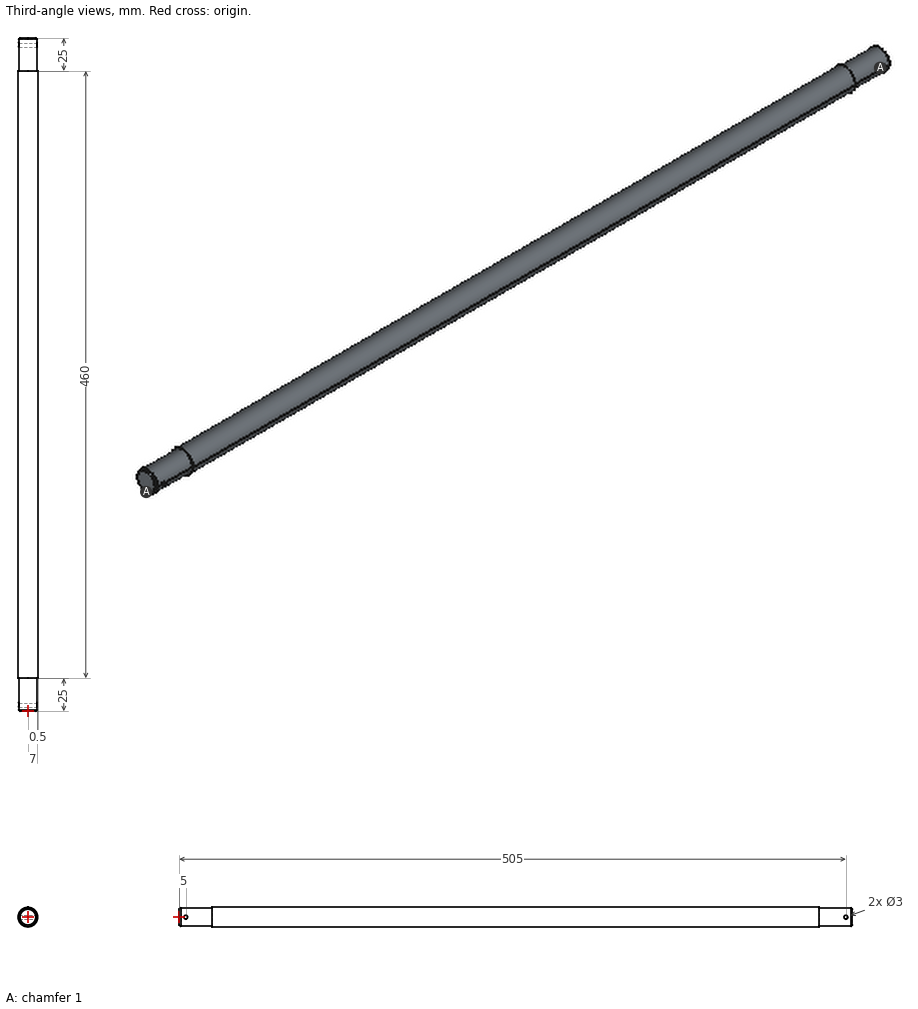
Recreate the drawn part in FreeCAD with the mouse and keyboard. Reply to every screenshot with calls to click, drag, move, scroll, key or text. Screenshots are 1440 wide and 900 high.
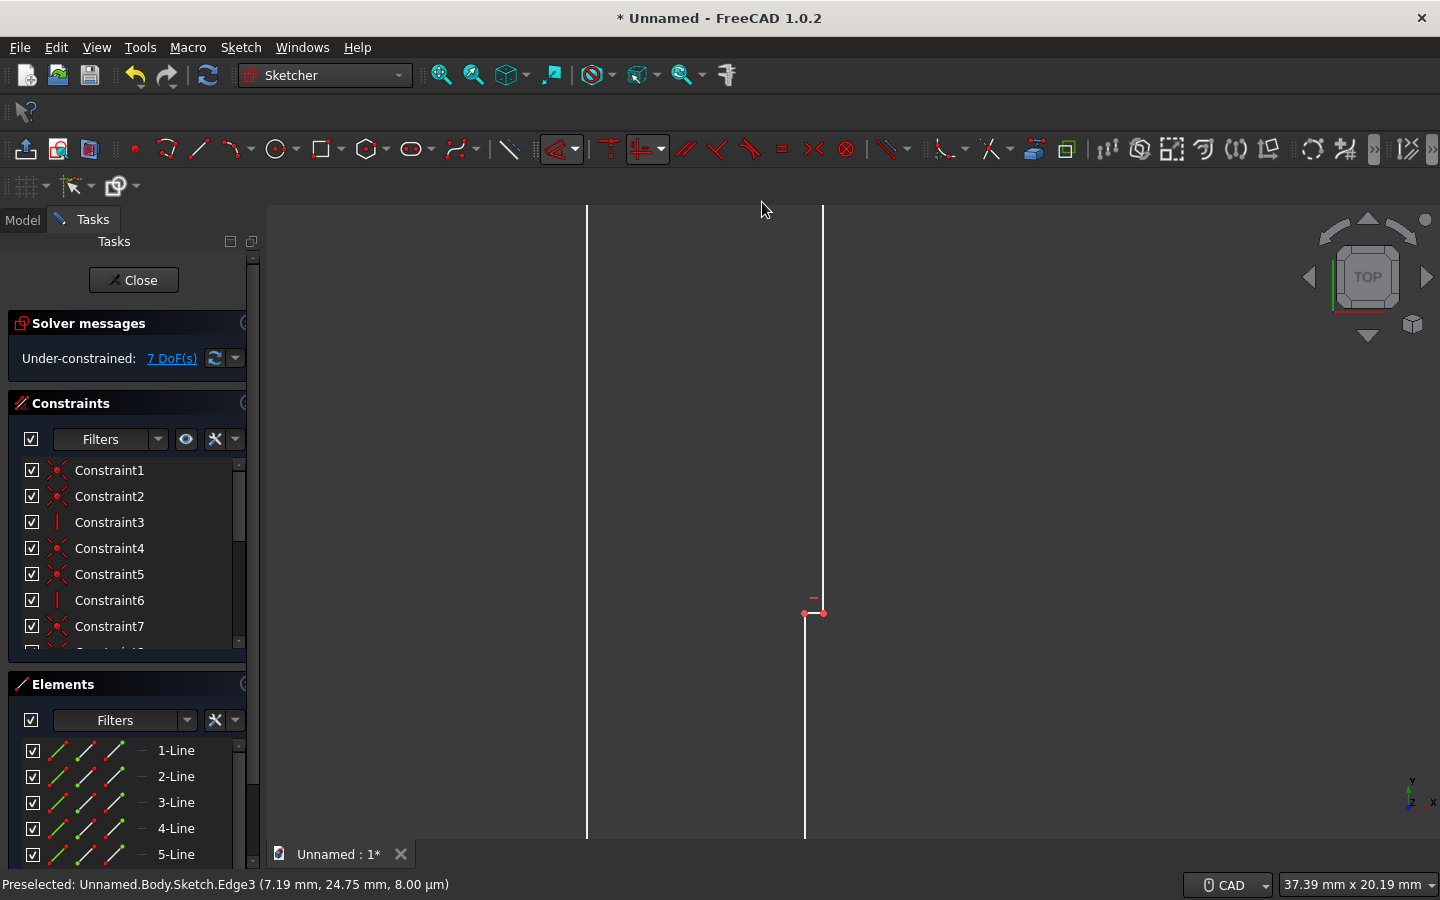
scroll(787, 723, down, 18)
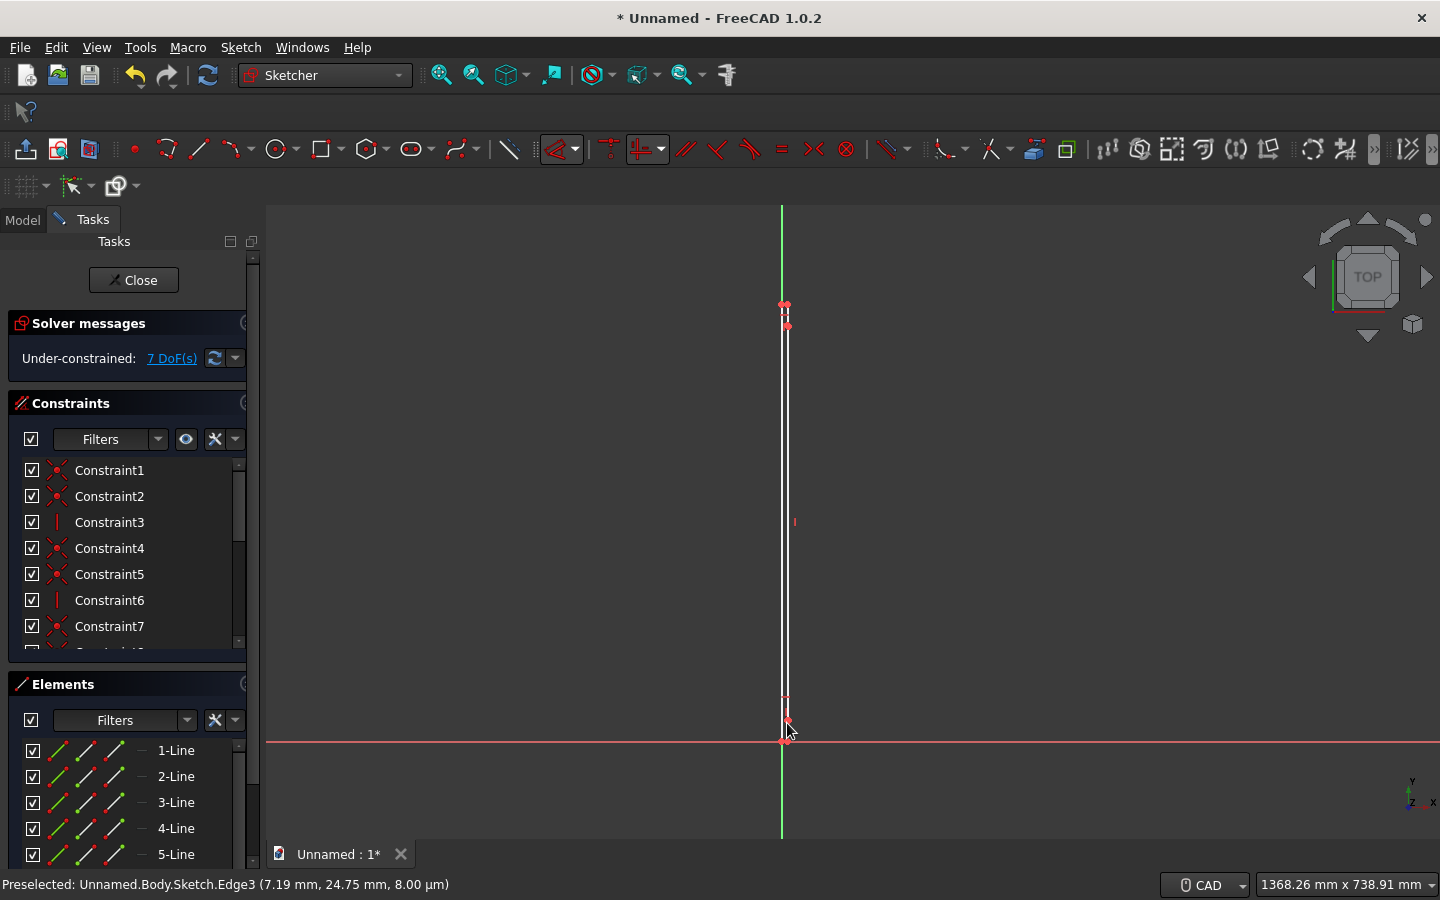
scroll(788, 326, up, 14)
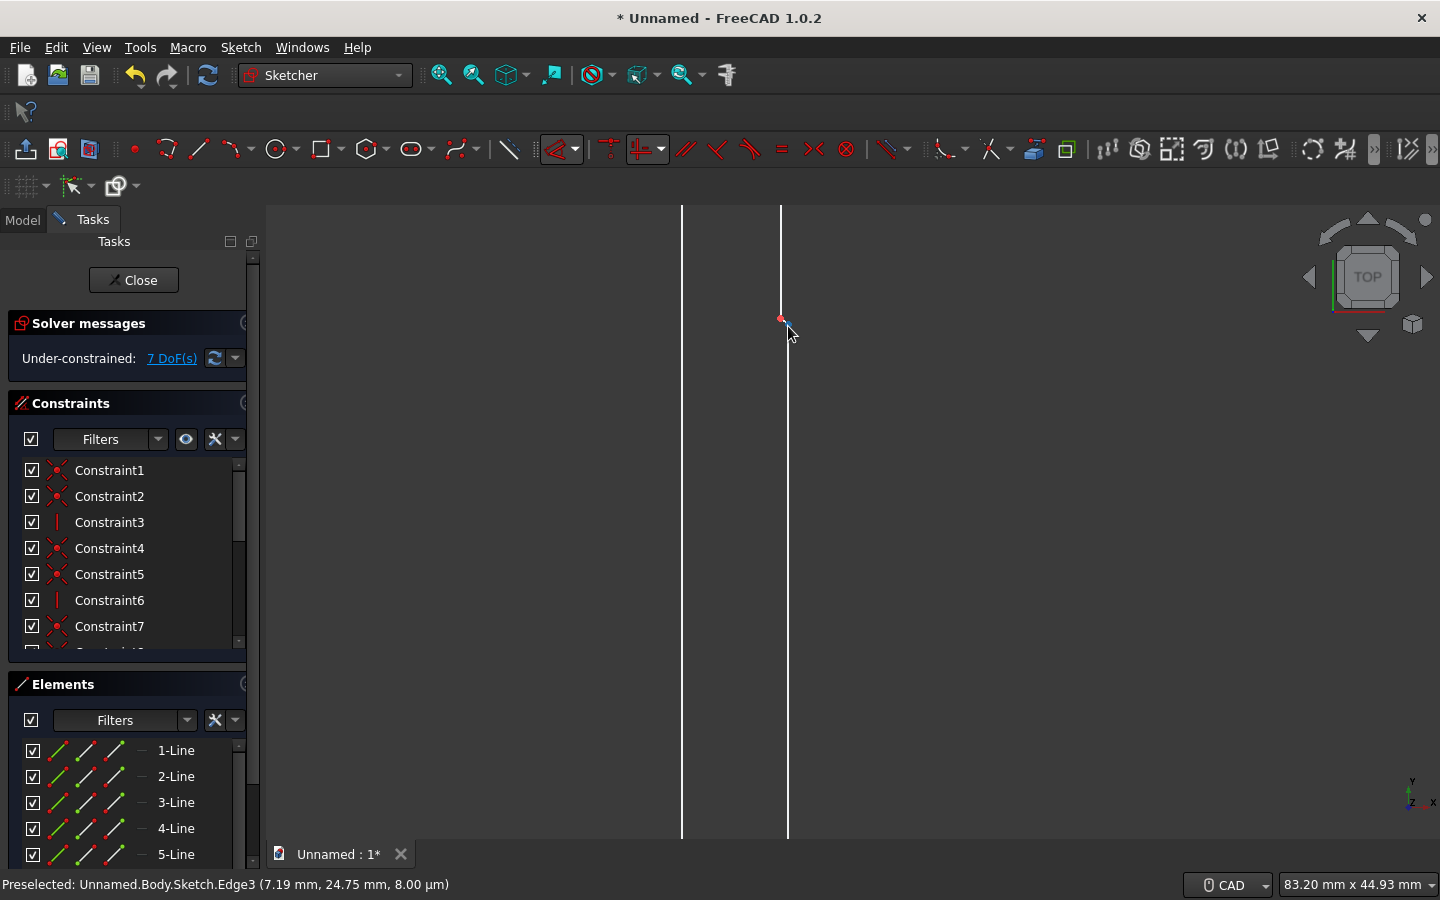
scroll(784, 321, up, 4)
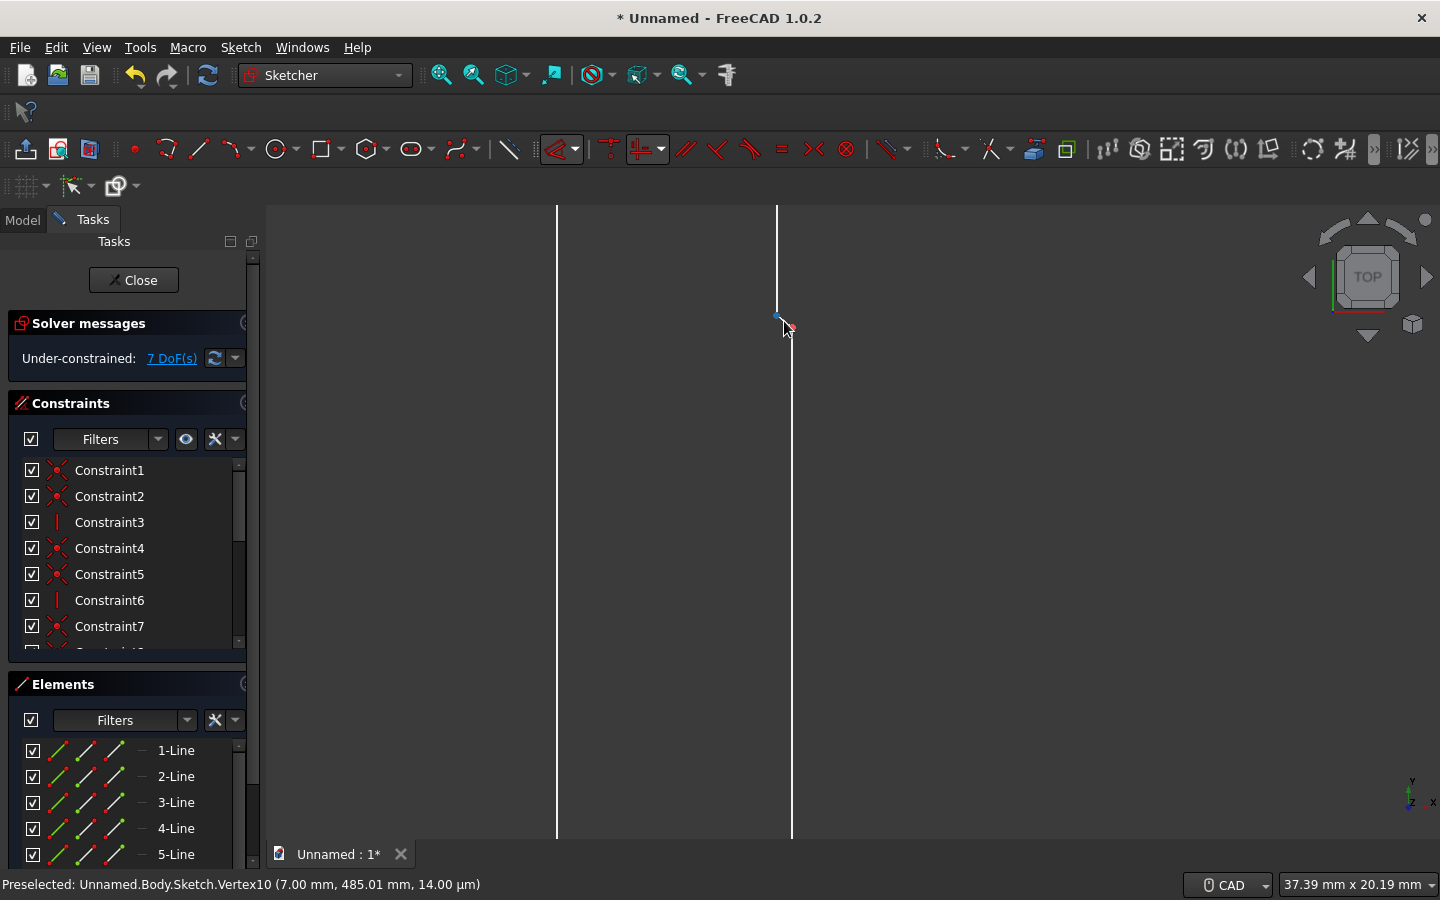
click(785, 321)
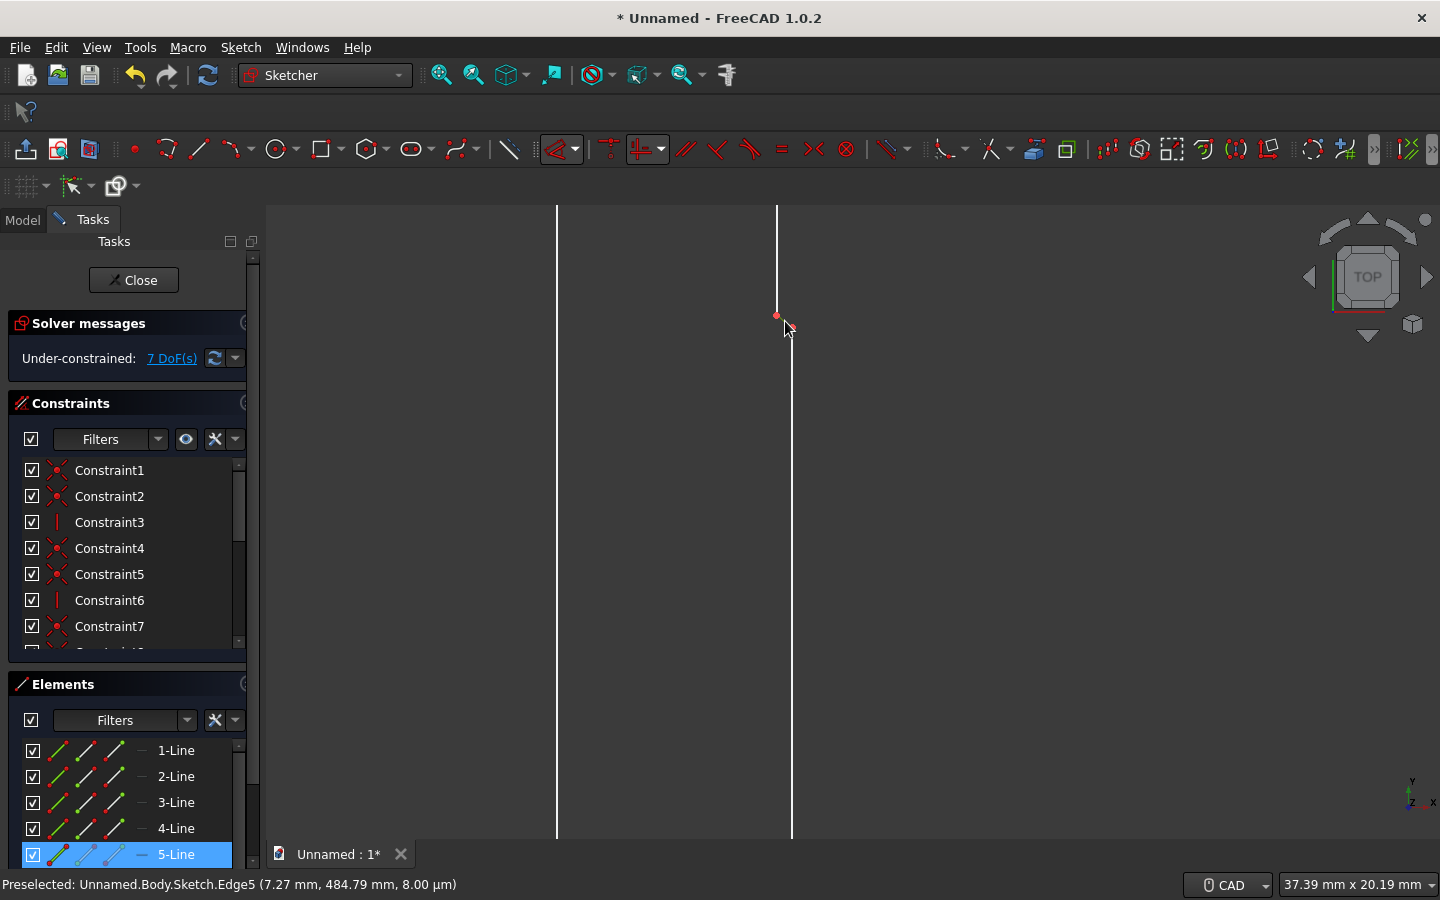
click(664, 150)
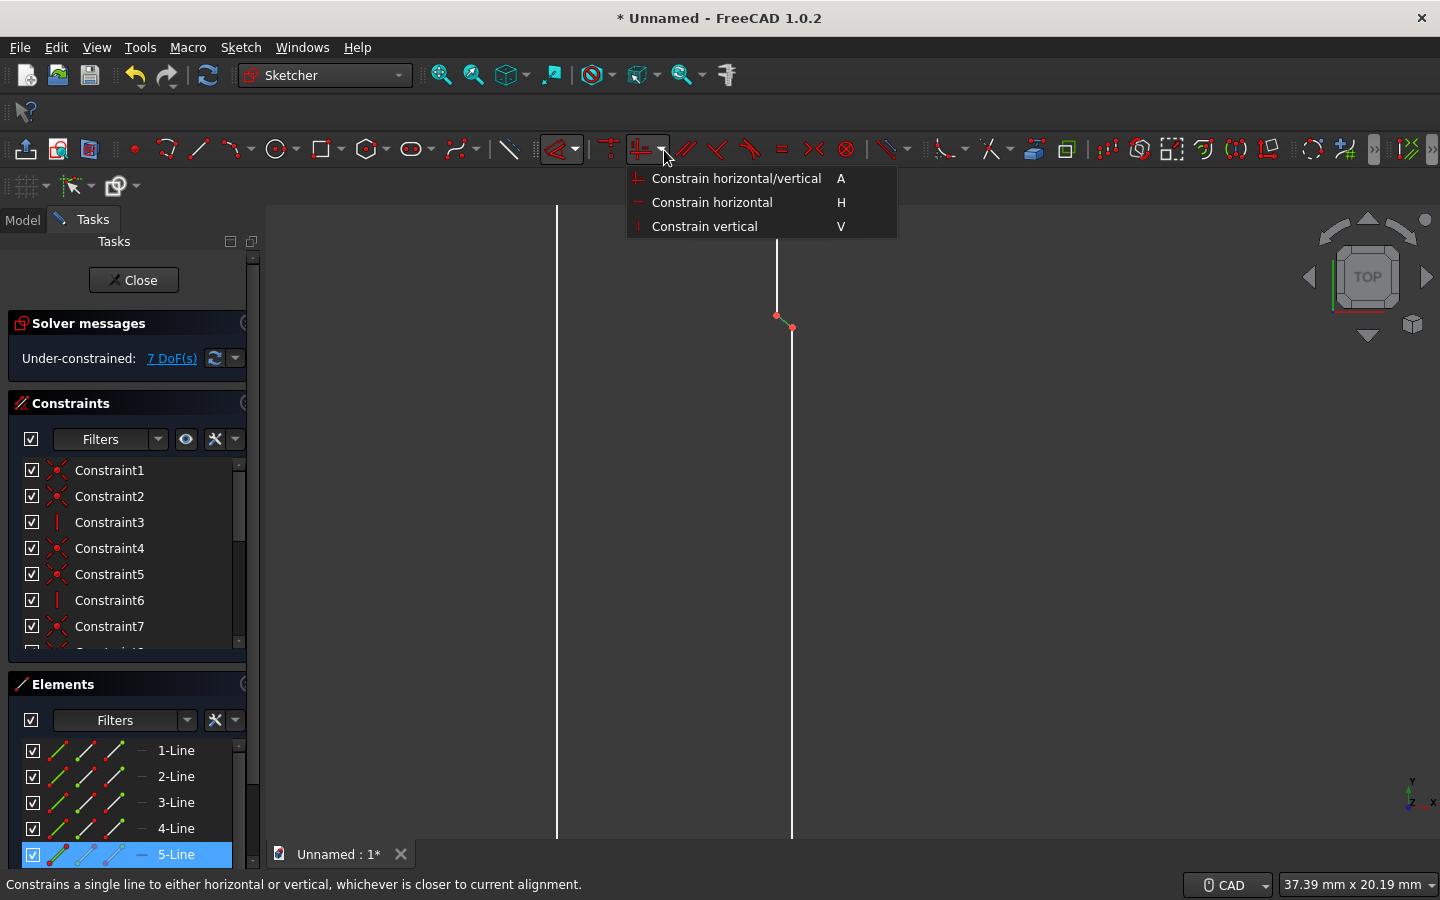
click(762, 202)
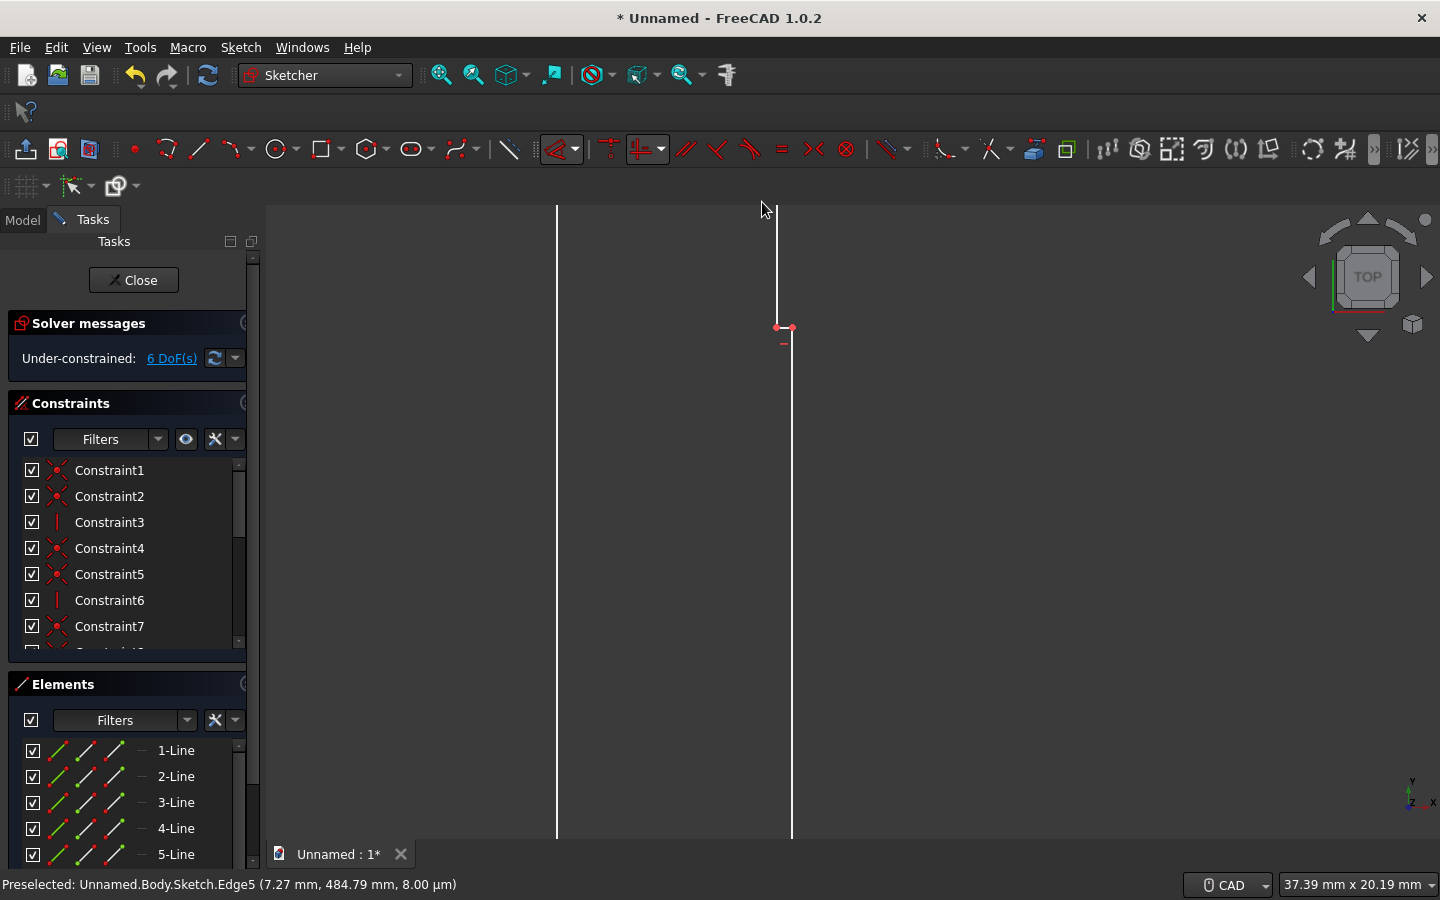
click(556, 150)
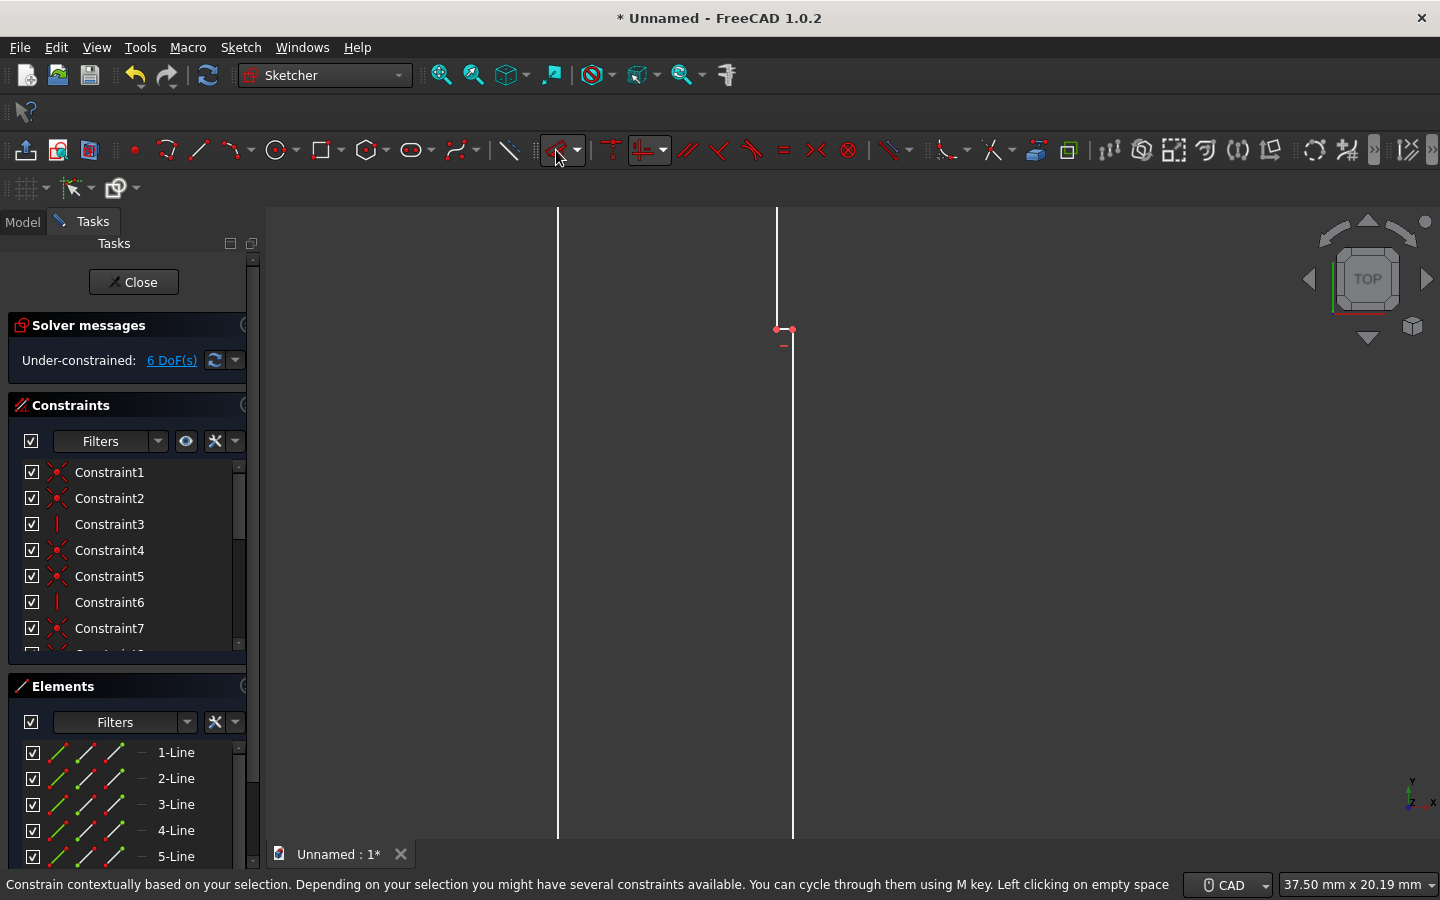
scroll(788, 327, down, 18)